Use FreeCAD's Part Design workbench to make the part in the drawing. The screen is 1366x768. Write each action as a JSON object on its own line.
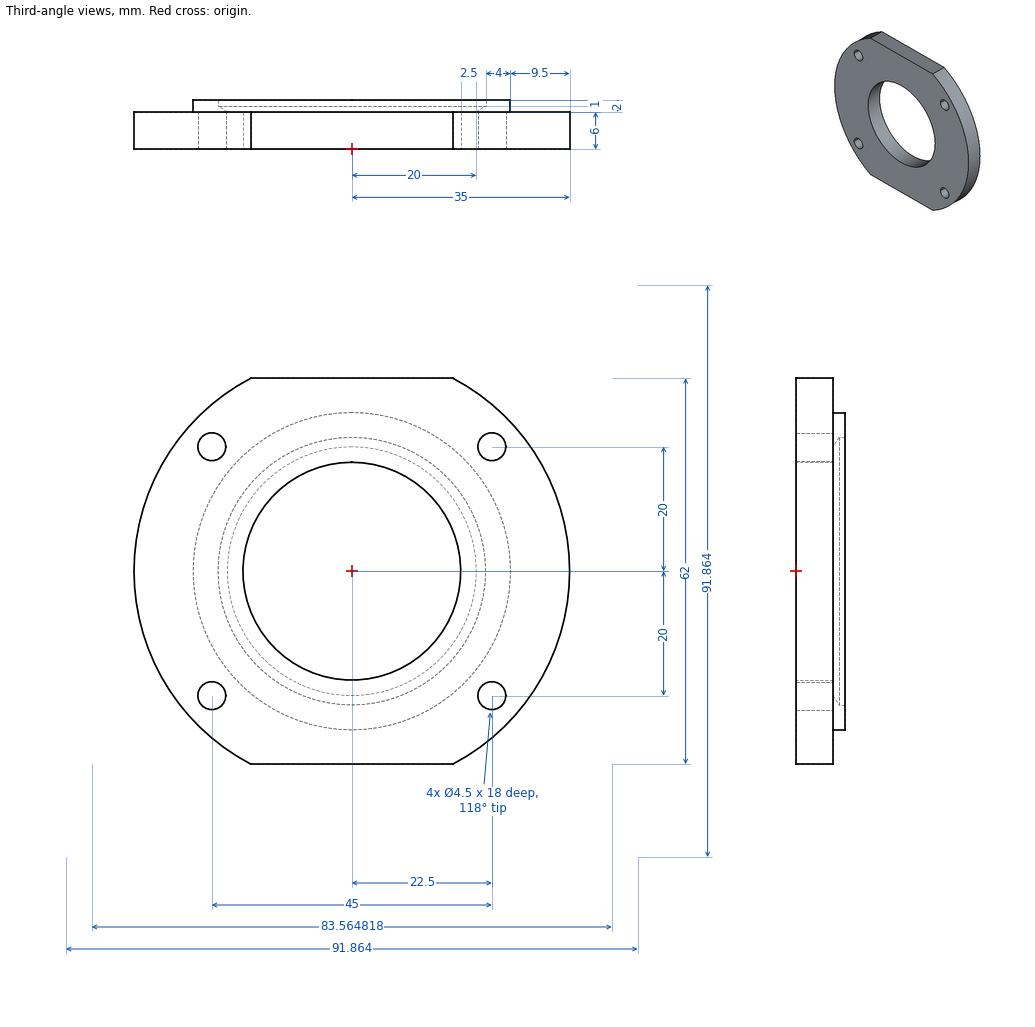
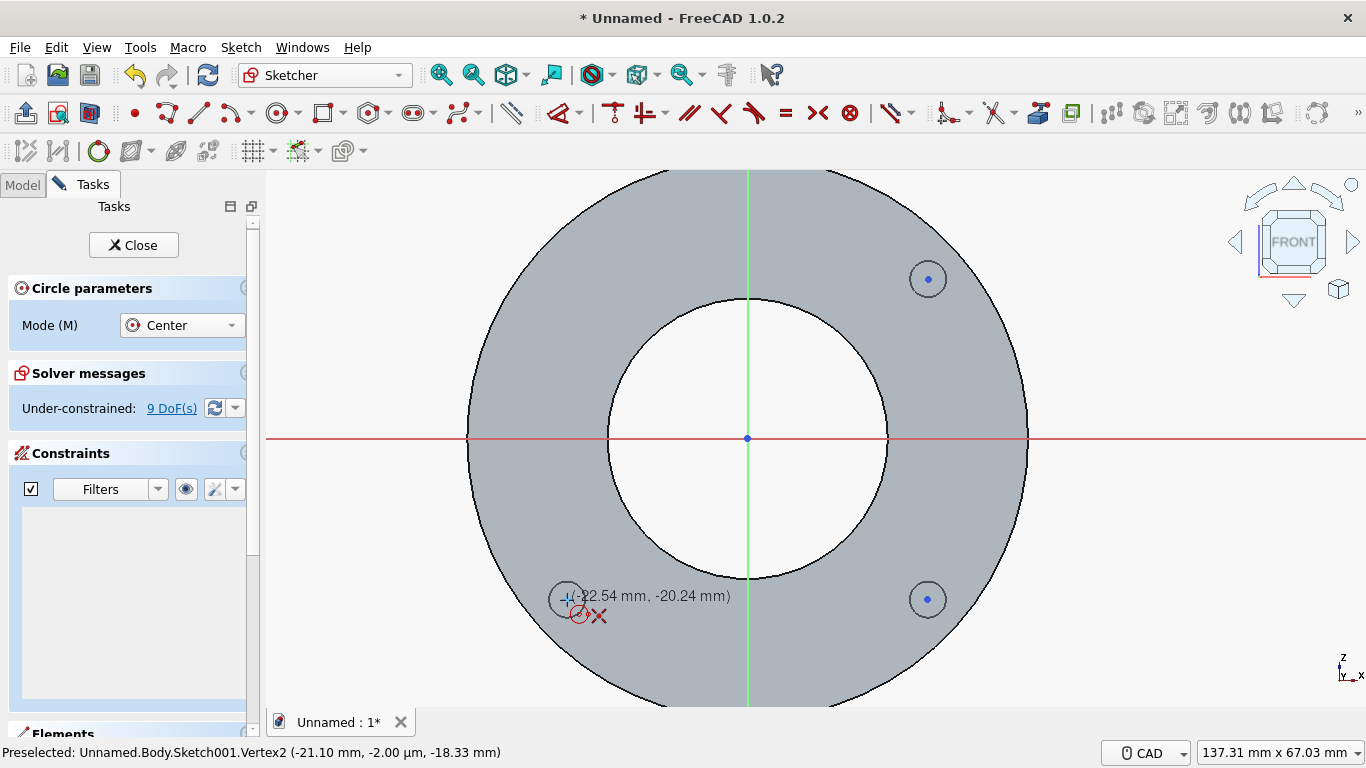
{"action": "scroll", "coordinate": [567, 279], "scroll_direction": "up", "scroll_amount": 2}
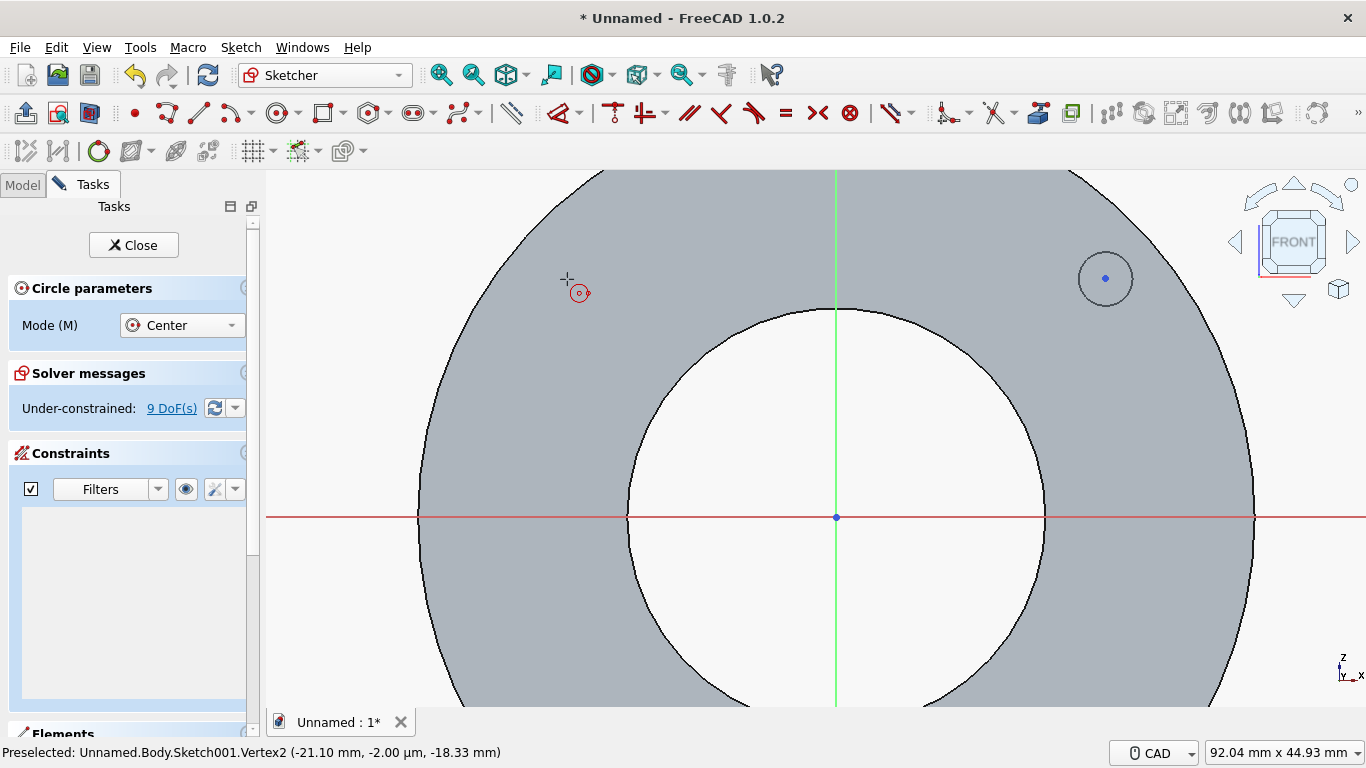
{"action": "left_click", "coordinate": [567, 278]}
{"action": "left_click", "coordinate": [586, 259]}
{"action": "key", "text": "Escape"}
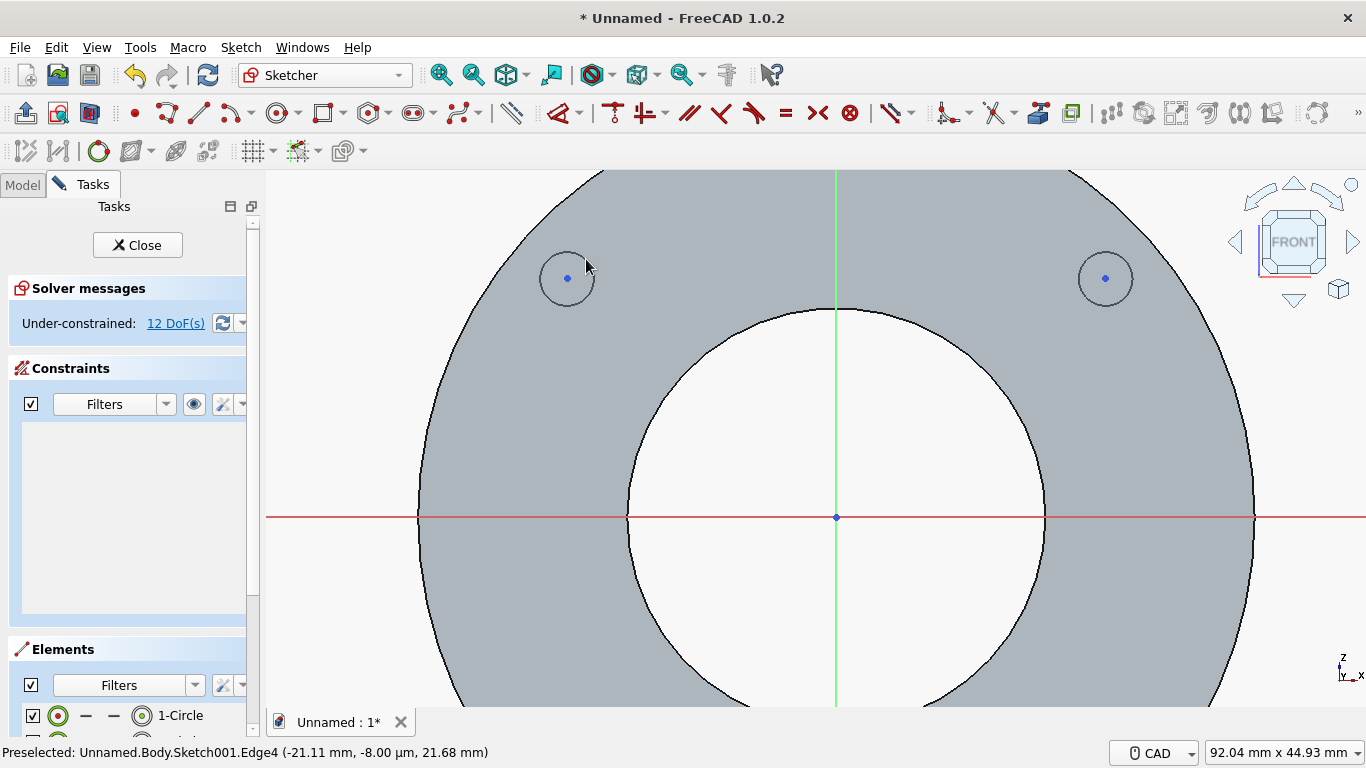
{"action": "scroll", "coordinate": [567, 278], "scroll_direction": "down", "scroll_amount": 2}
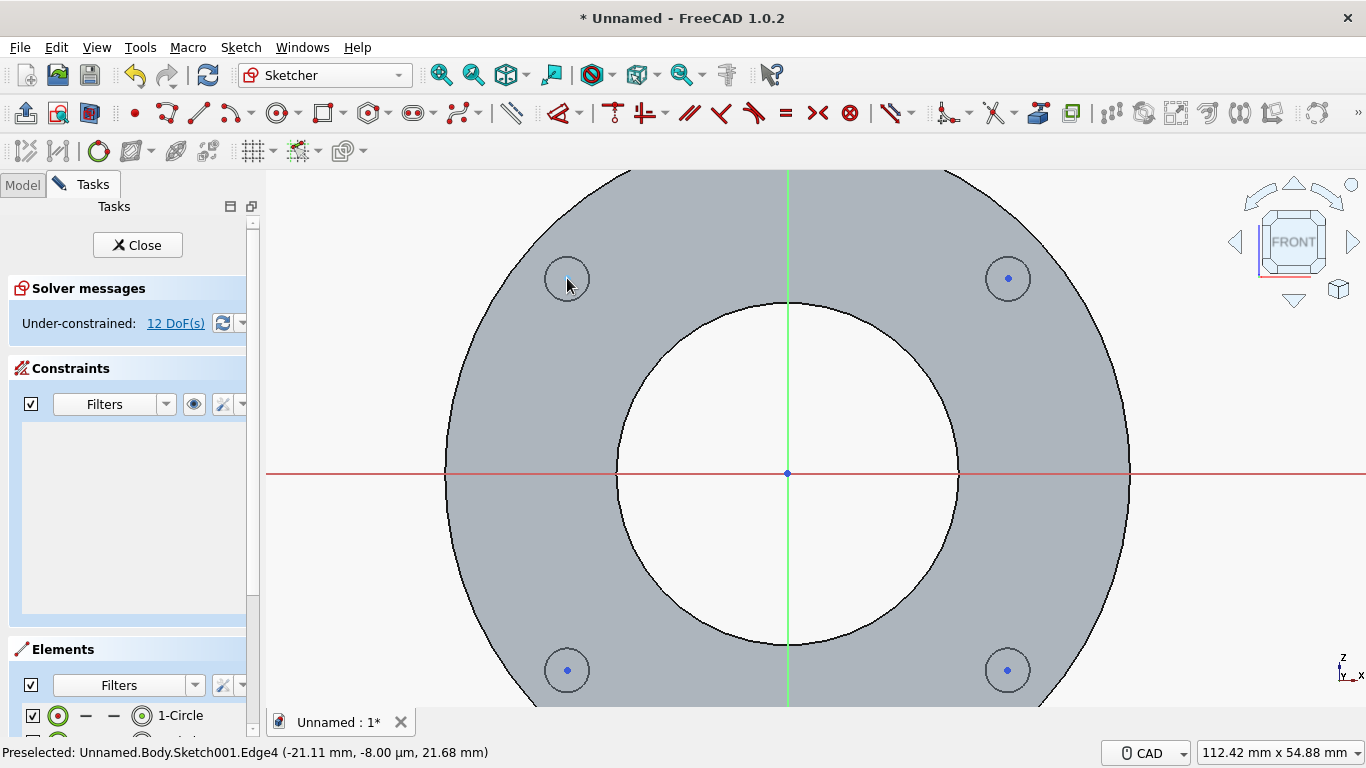
{"action": "left_click", "coordinate": [941, 586]}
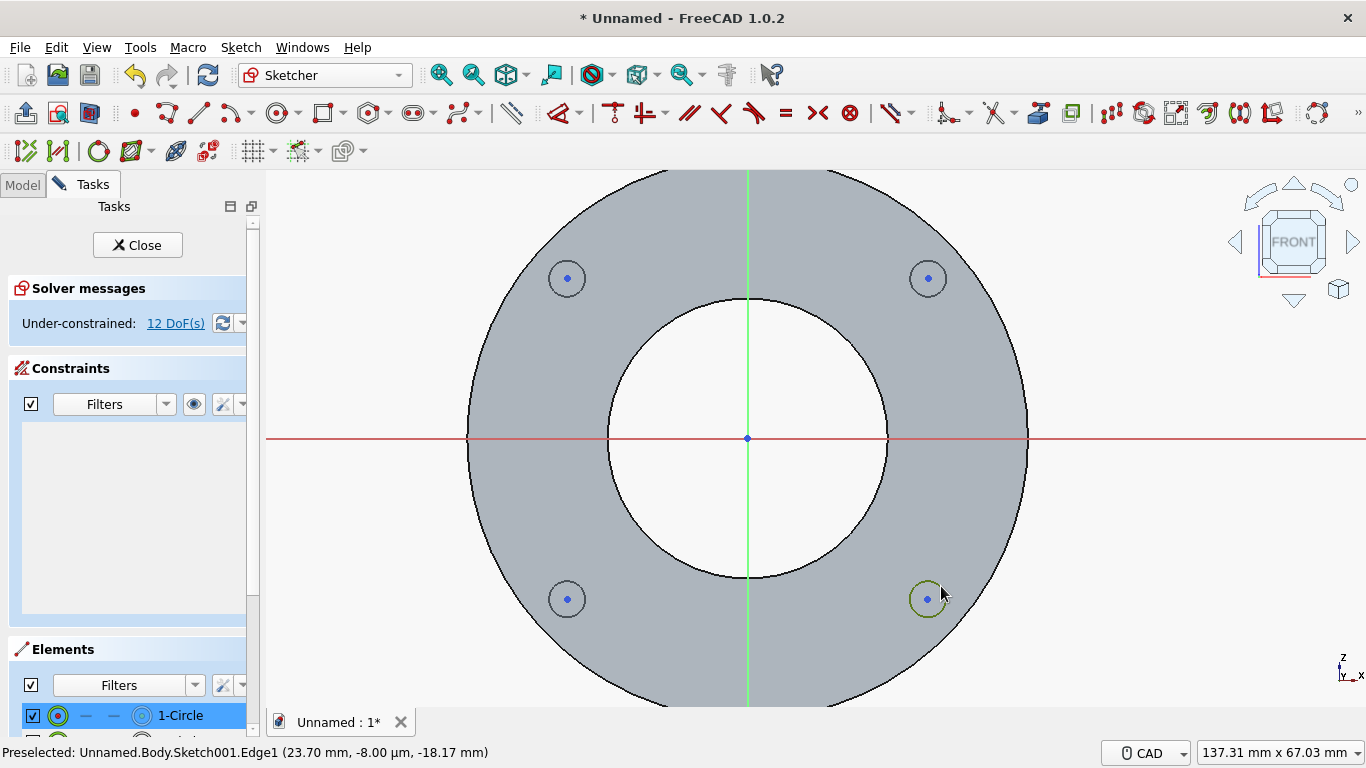
{"action": "left_click", "coordinate": [941, 266]}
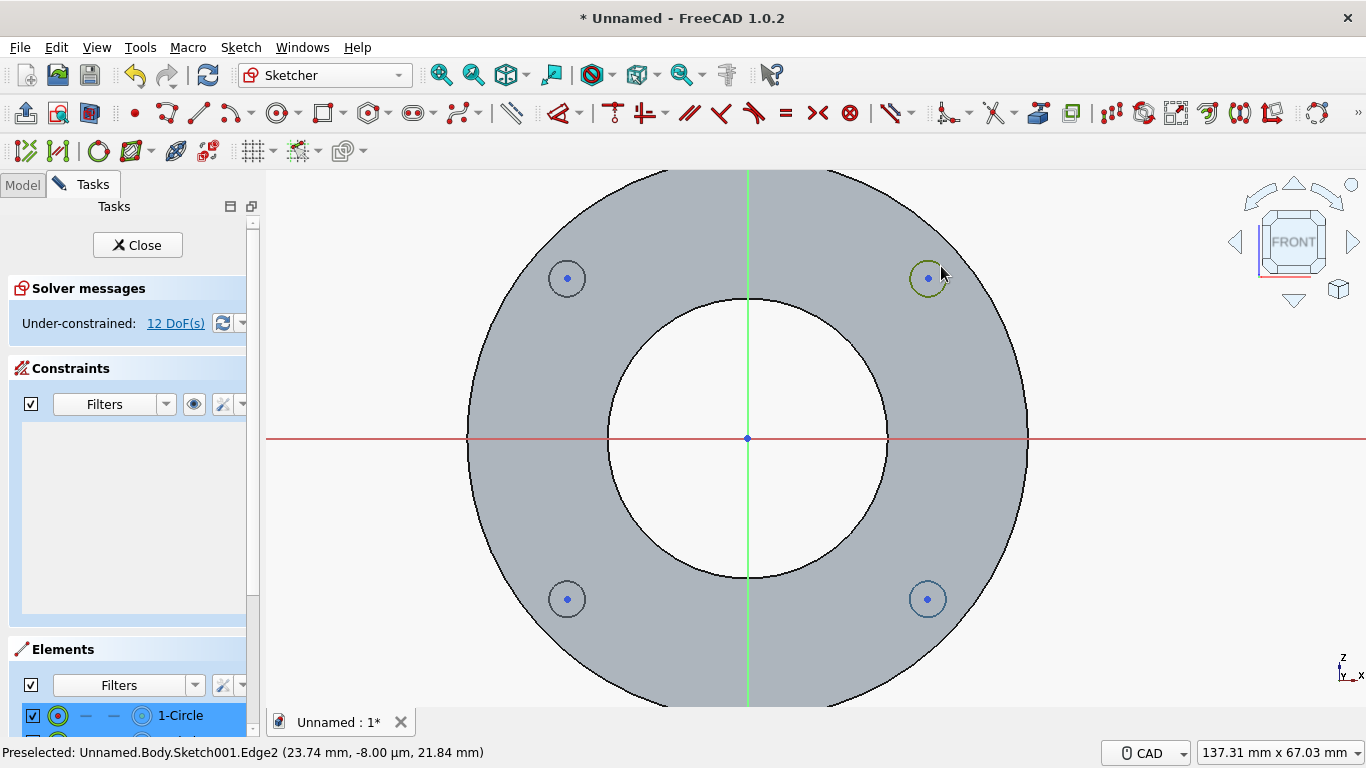
{"action": "left_click", "coordinate": [580, 586]}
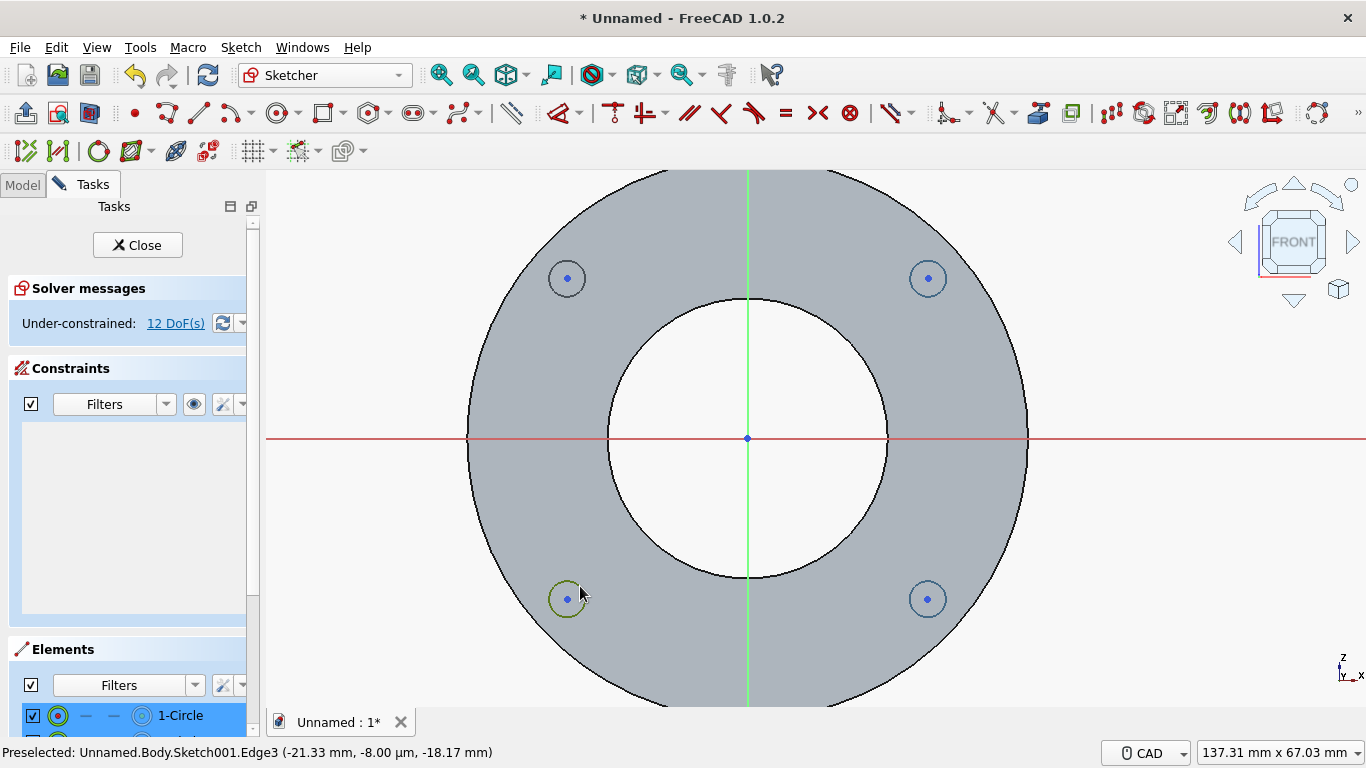
{"action": "left_click", "coordinate": [580, 266]}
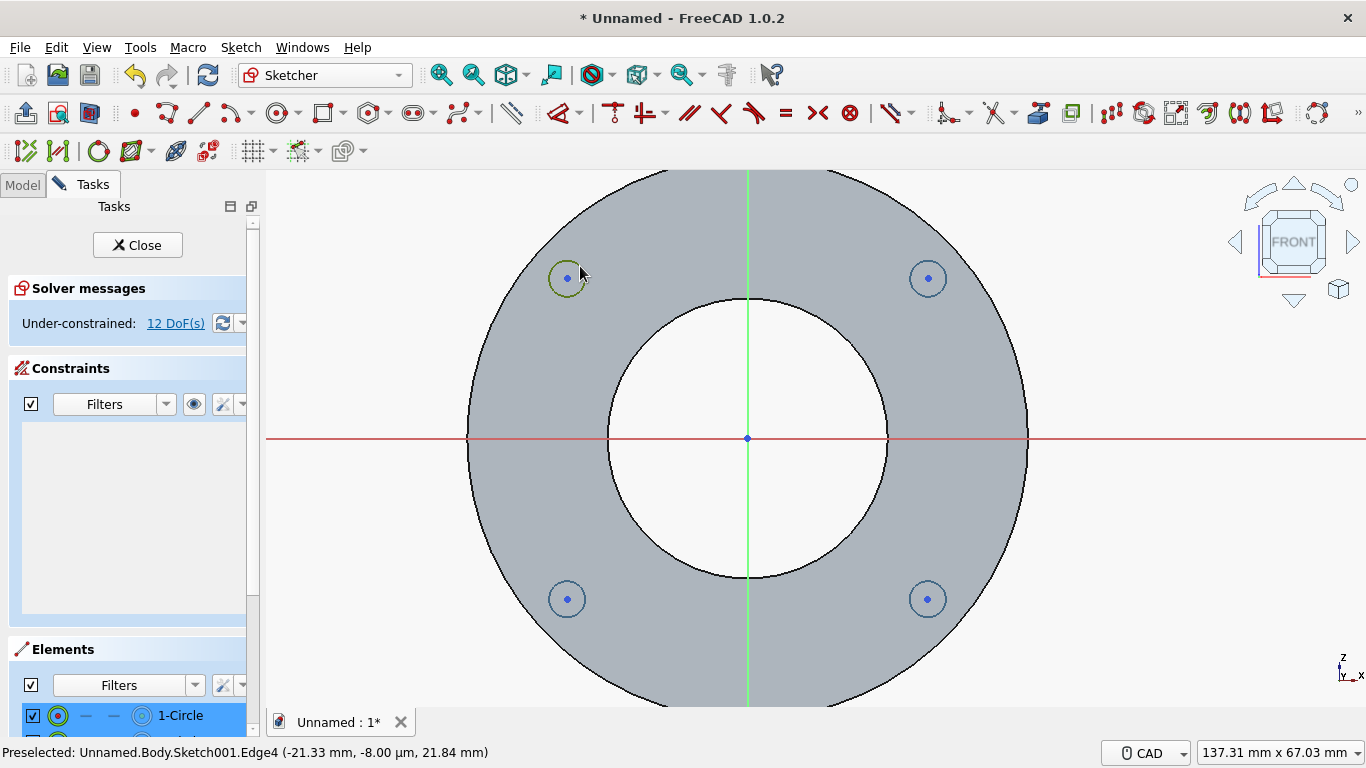
{"action": "left_click", "coordinate": [786, 114]}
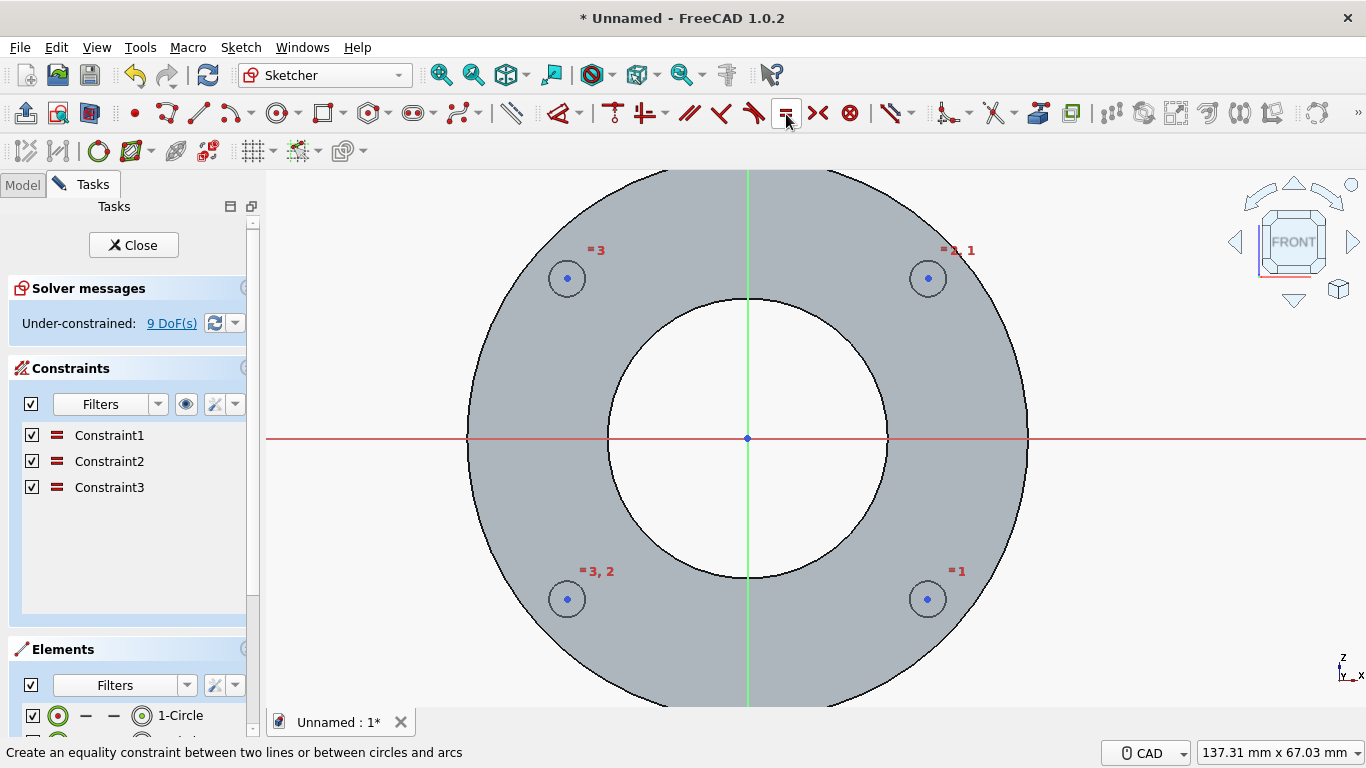
{"action": "left_click", "coordinate": [928, 599]}